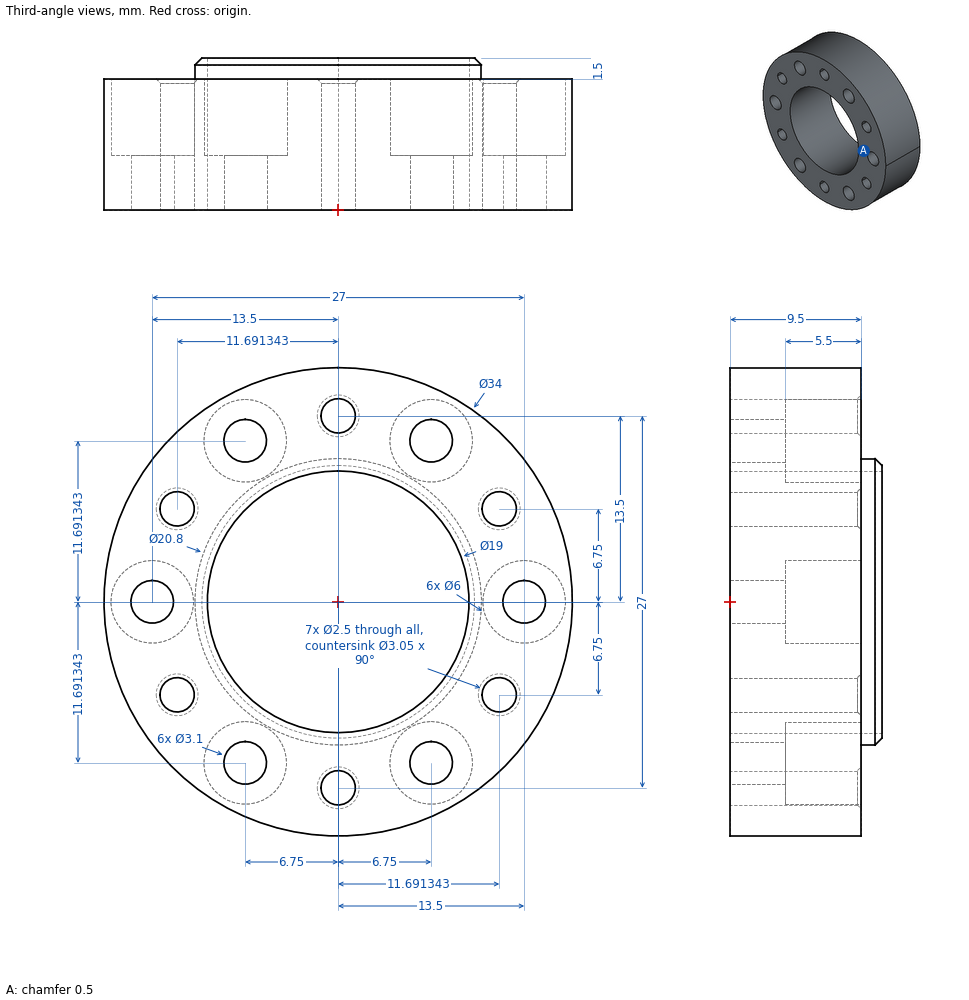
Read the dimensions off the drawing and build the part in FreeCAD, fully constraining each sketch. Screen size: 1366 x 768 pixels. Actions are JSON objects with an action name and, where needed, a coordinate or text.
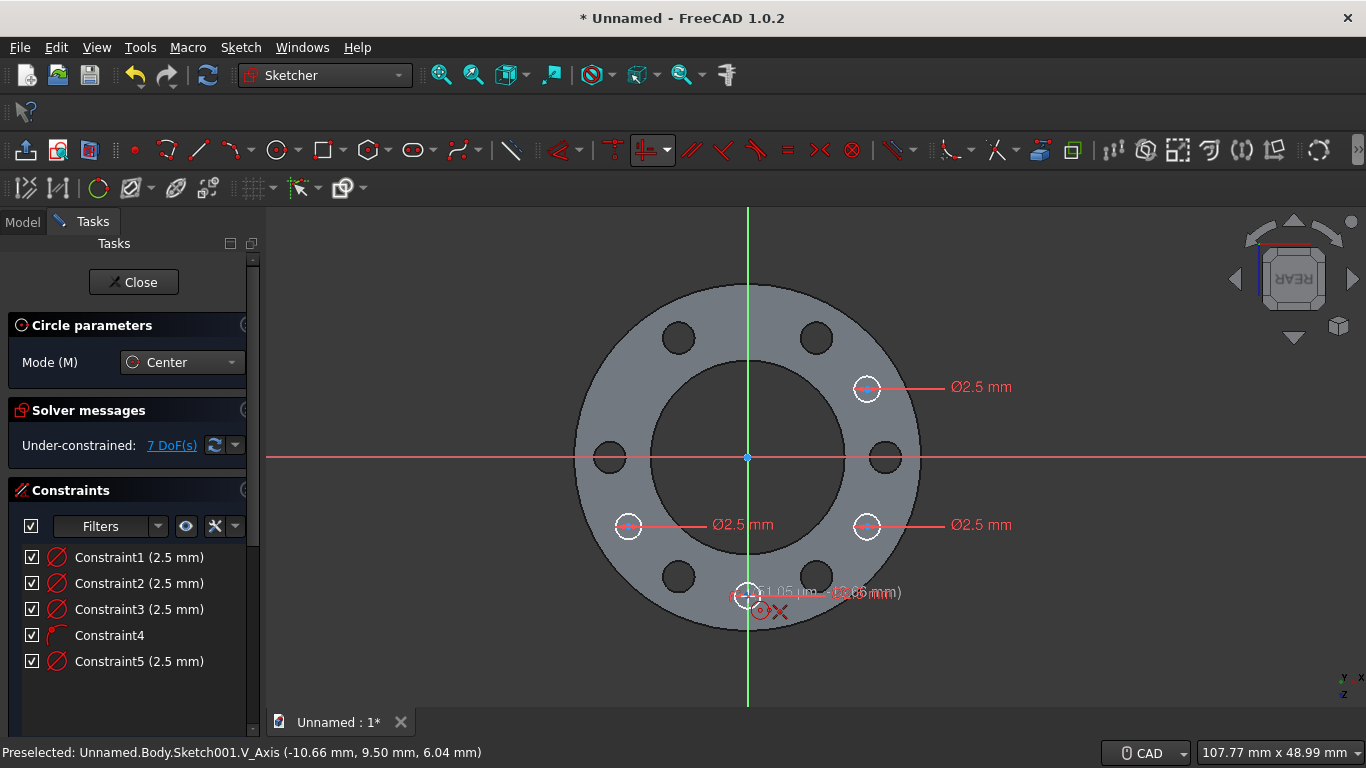
{"action": "scroll", "coordinate": [628, 389], "scroll_direction": "up", "scroll_amount": 3}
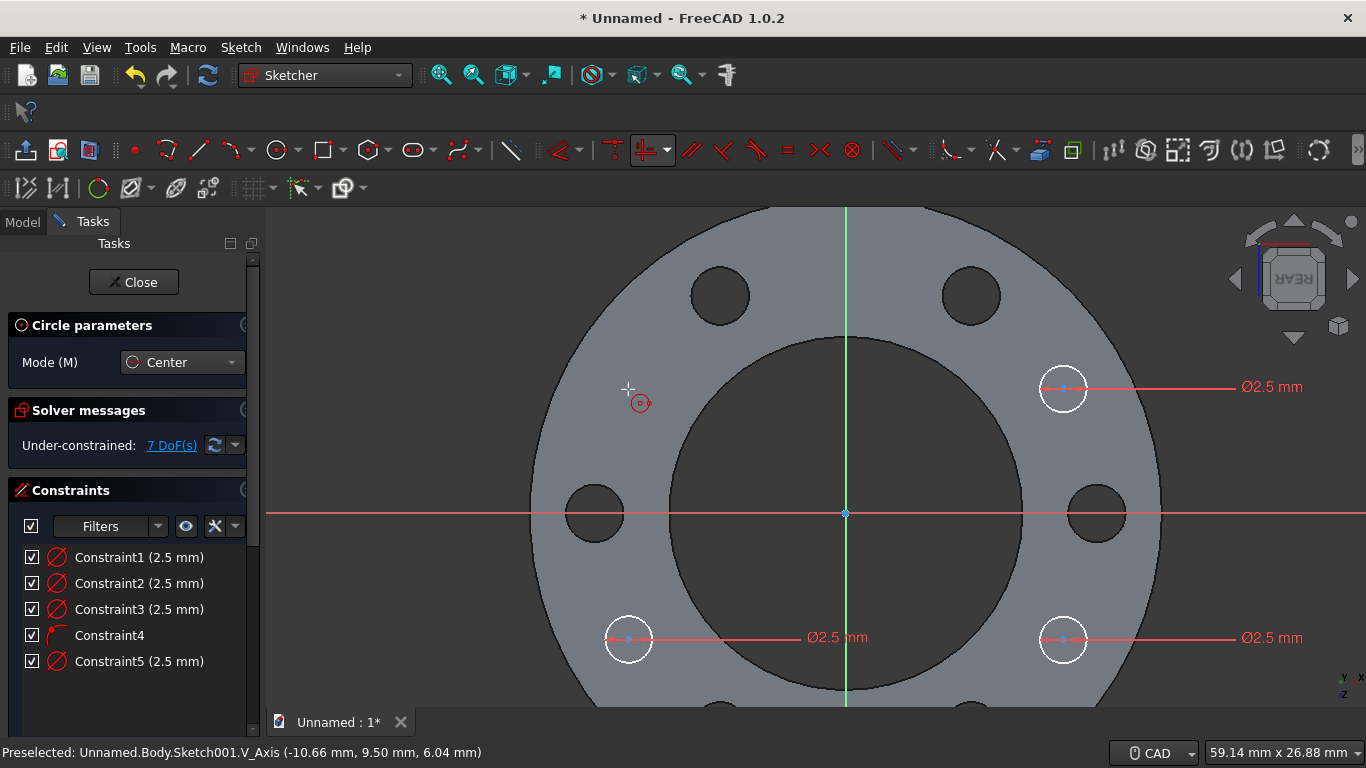
{"action": "left_click", "coordinate": [628, 388]}
{"action": "mouse_move", "coordinate": [645, 371]}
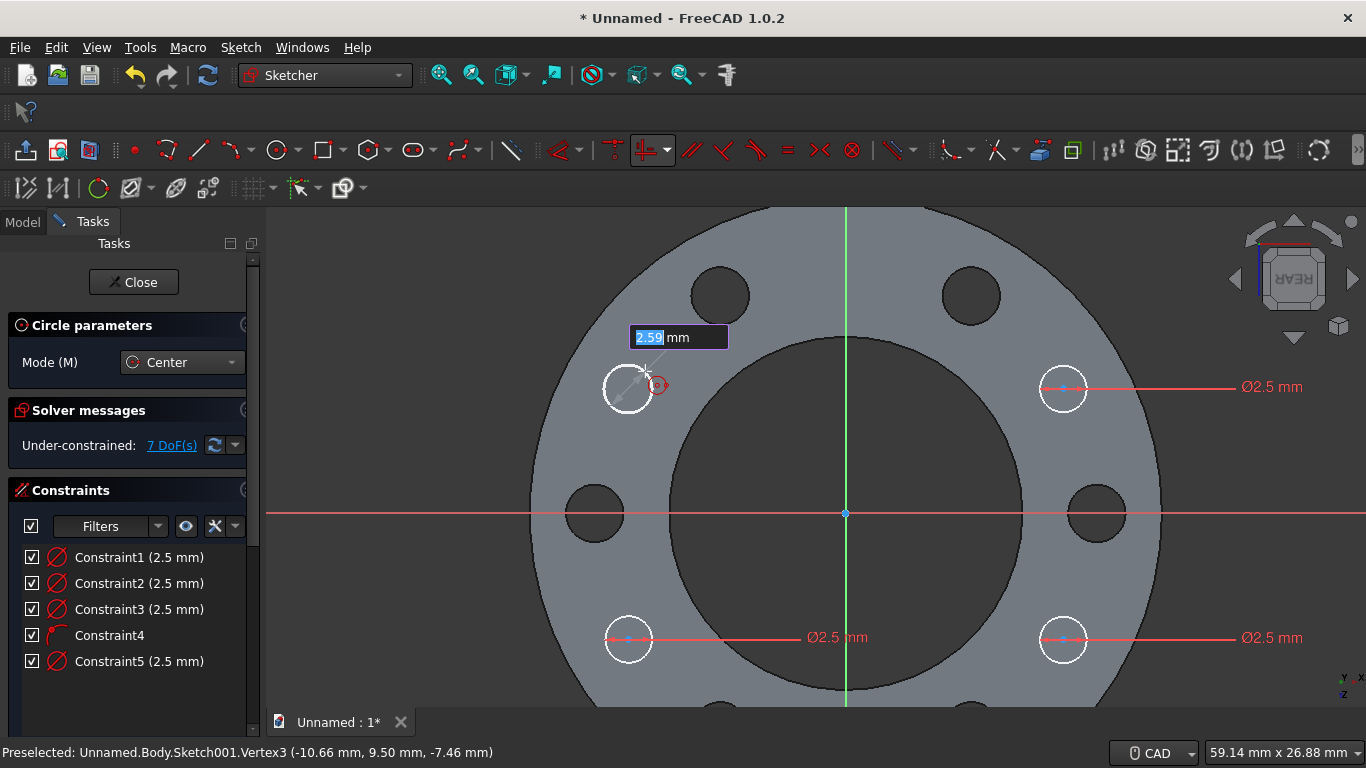
{"action": "type", "text": "2.5"}
{"action": "key", "text": "Return"}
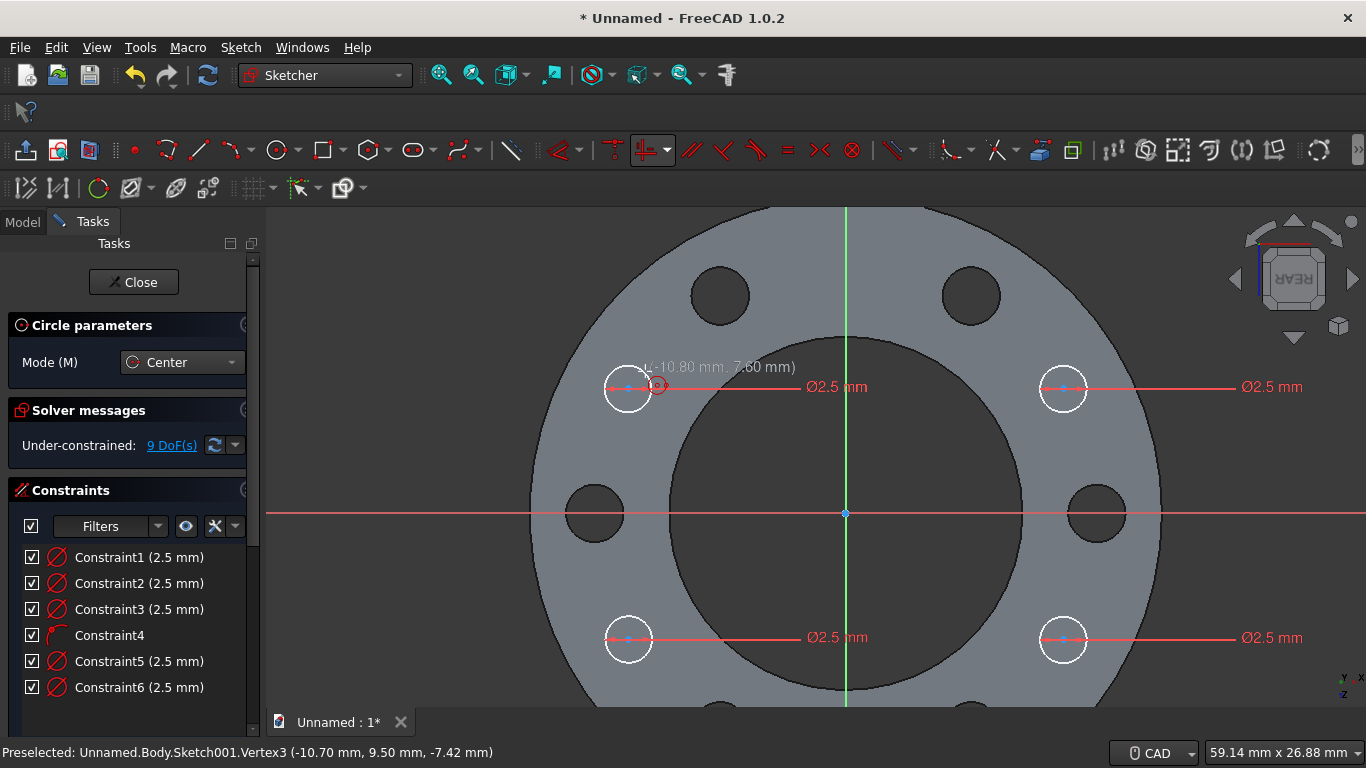
{"action": "left_click", "coordinate": [846, 262]}
{"action": "mouse_move", "coordinate": [862, 246]}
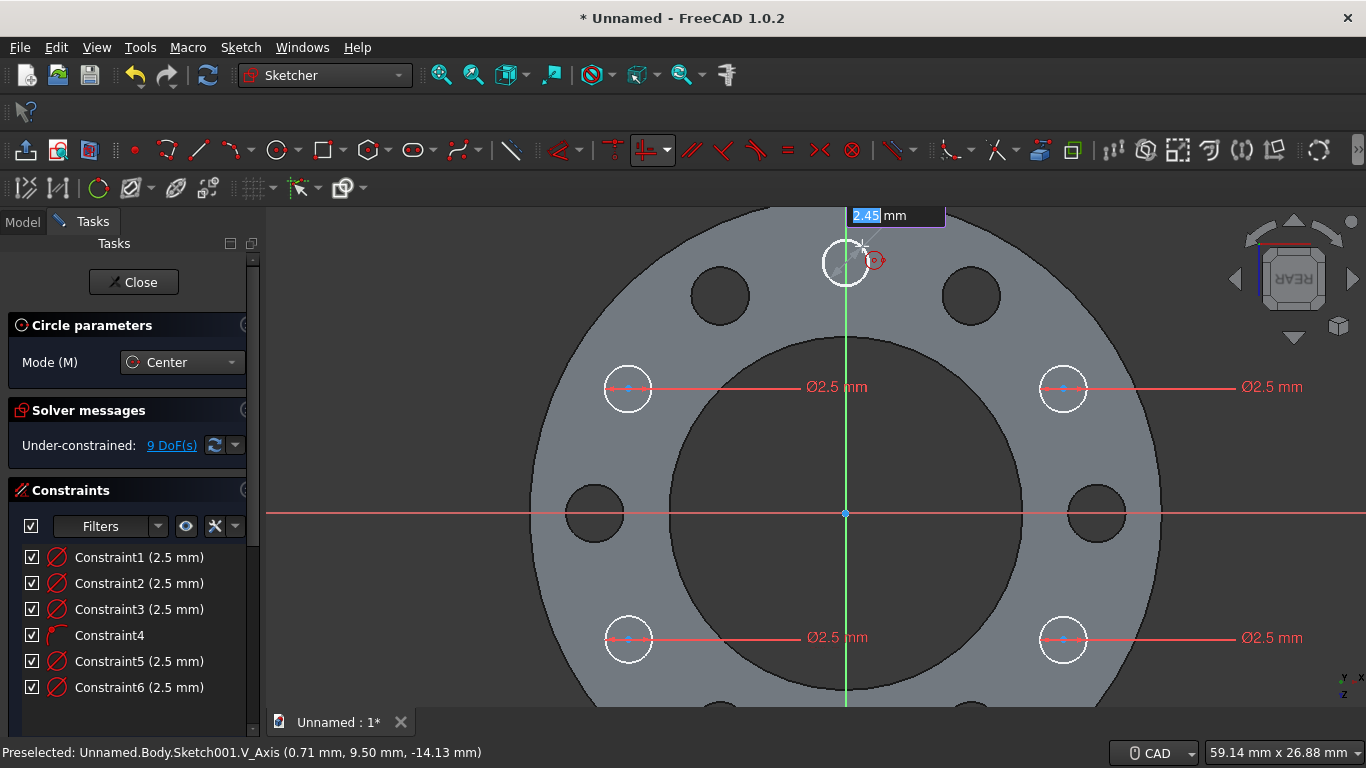
{"action": "type", "text": "2.5"}
{"action": "key", "text": "Return"}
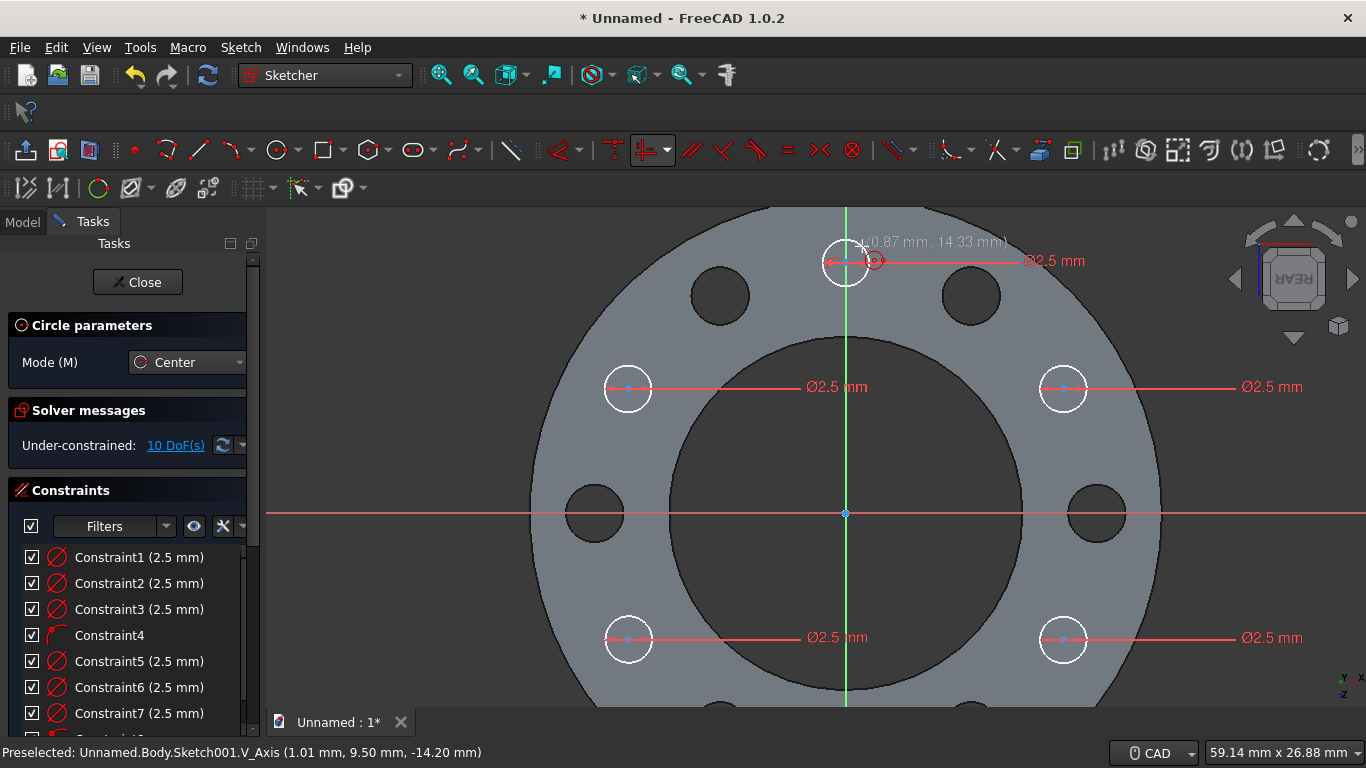
{"action": "left_click", "coordinate": [846, 513]}
{"action": "mouse_move", "coordinate": [862, 497]}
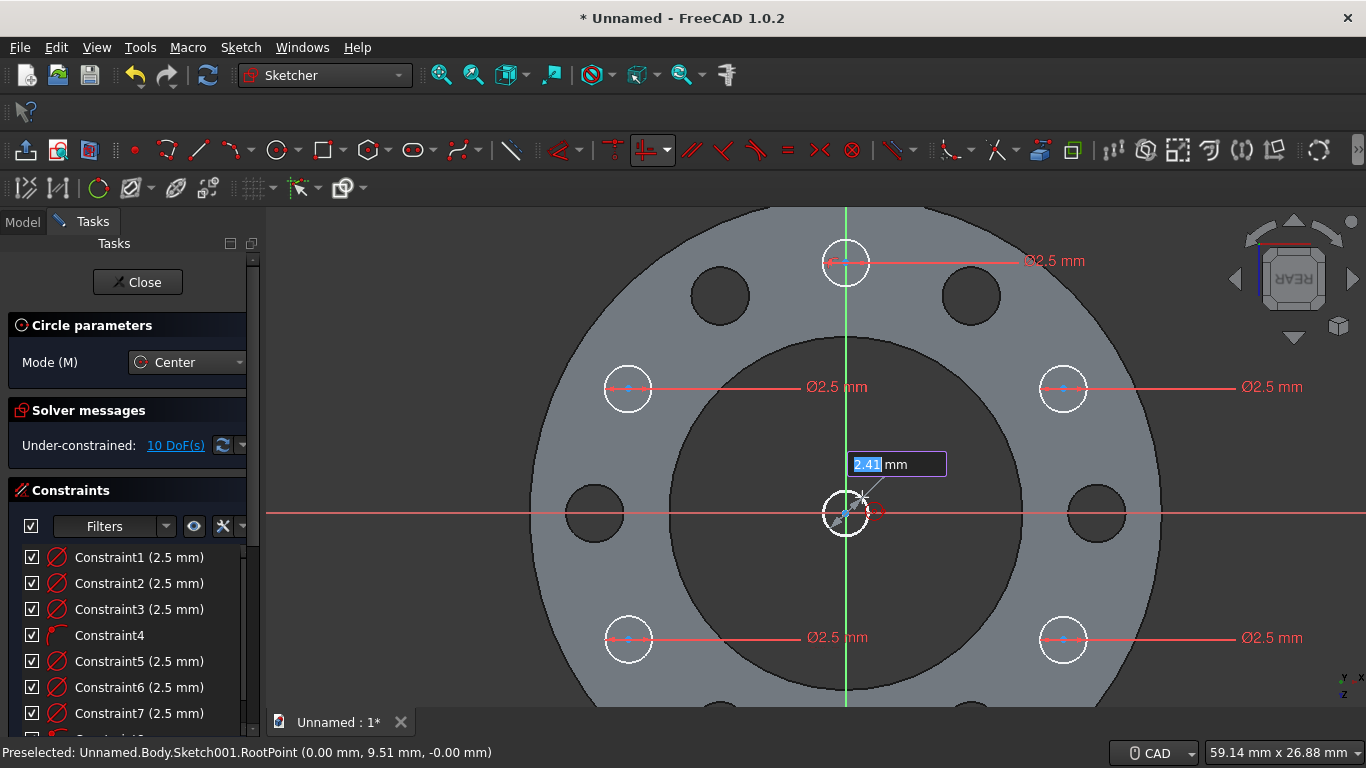
{"action": "type", "text": "2.5"}
{"action": "key", "text": "Return"}
{"action": "key", "text": "Escape"}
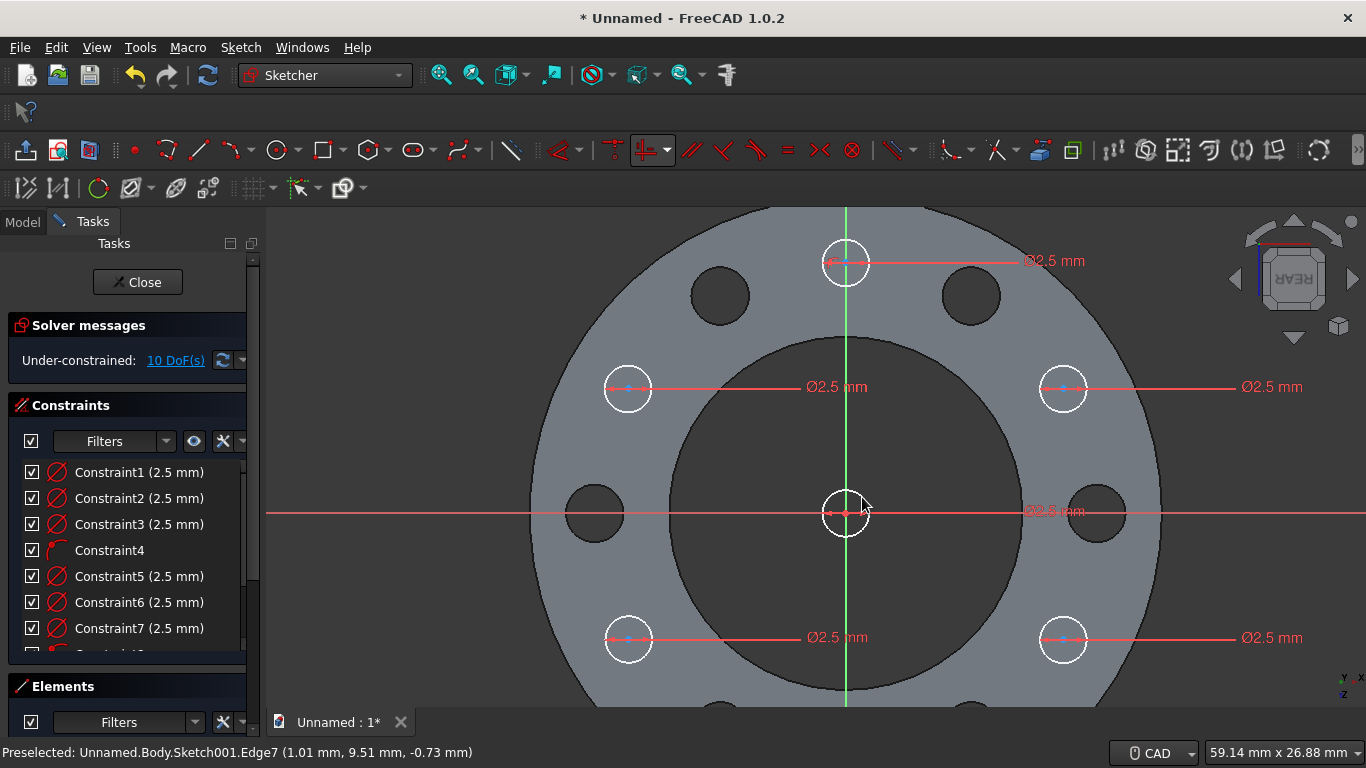
{"action": "left_click", "coordinate": [1063, 389]}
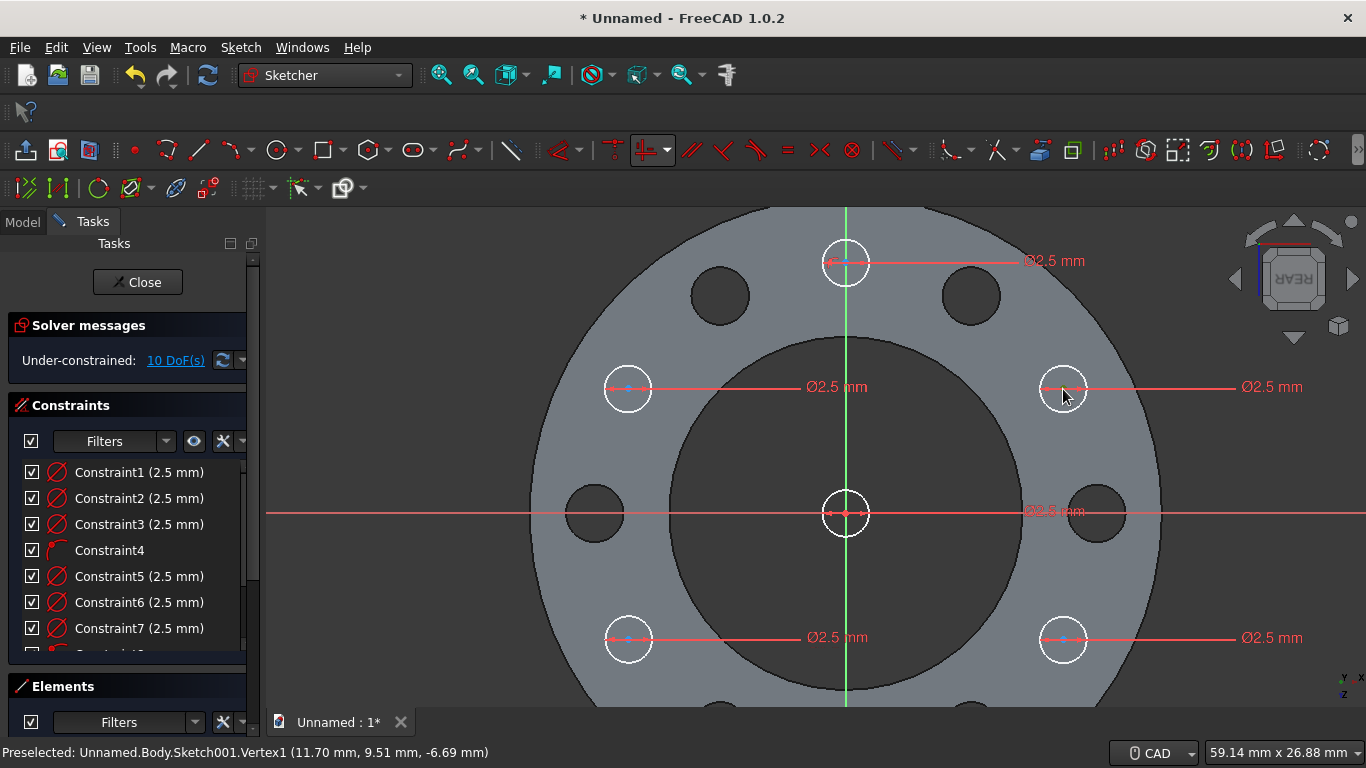
{"action": "left_click", "coordinate": [1063, 640]}